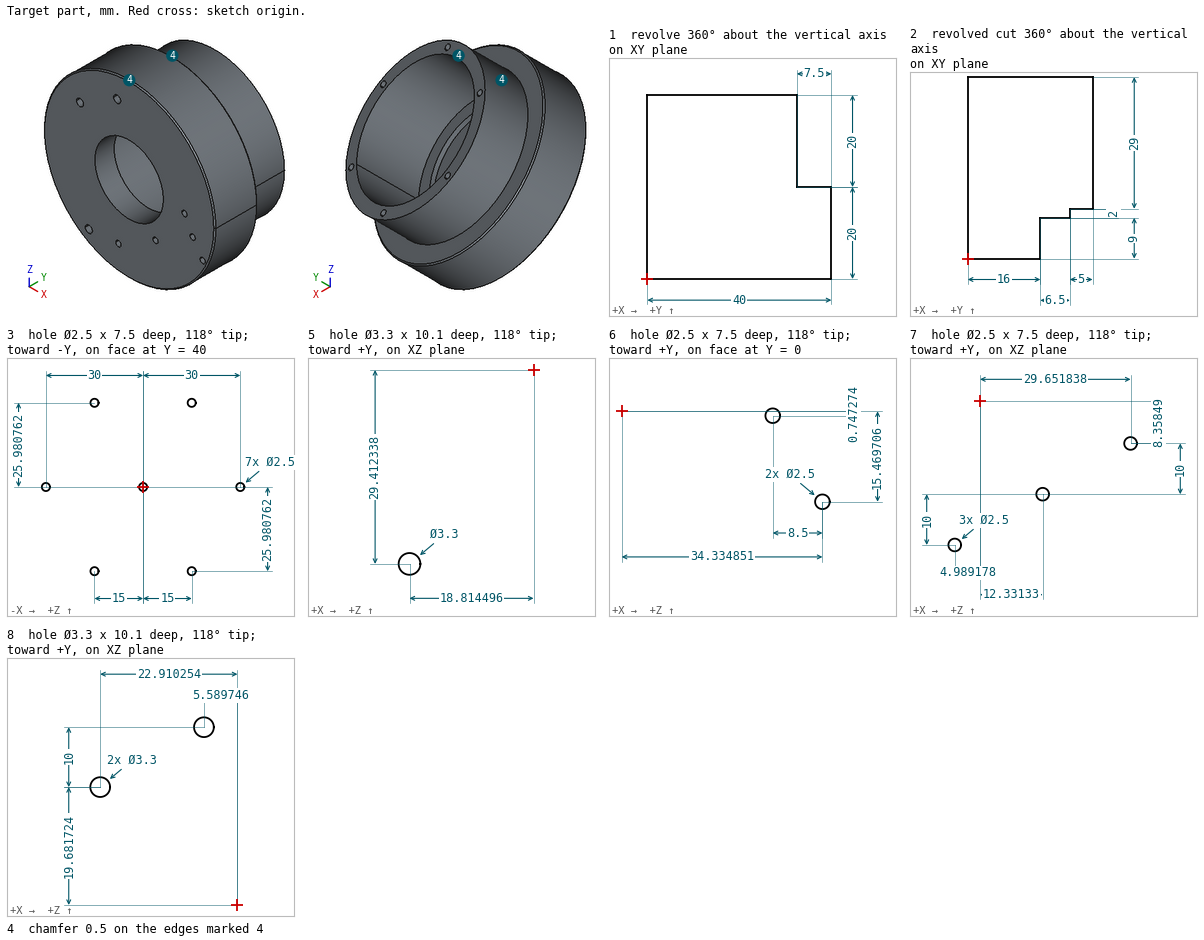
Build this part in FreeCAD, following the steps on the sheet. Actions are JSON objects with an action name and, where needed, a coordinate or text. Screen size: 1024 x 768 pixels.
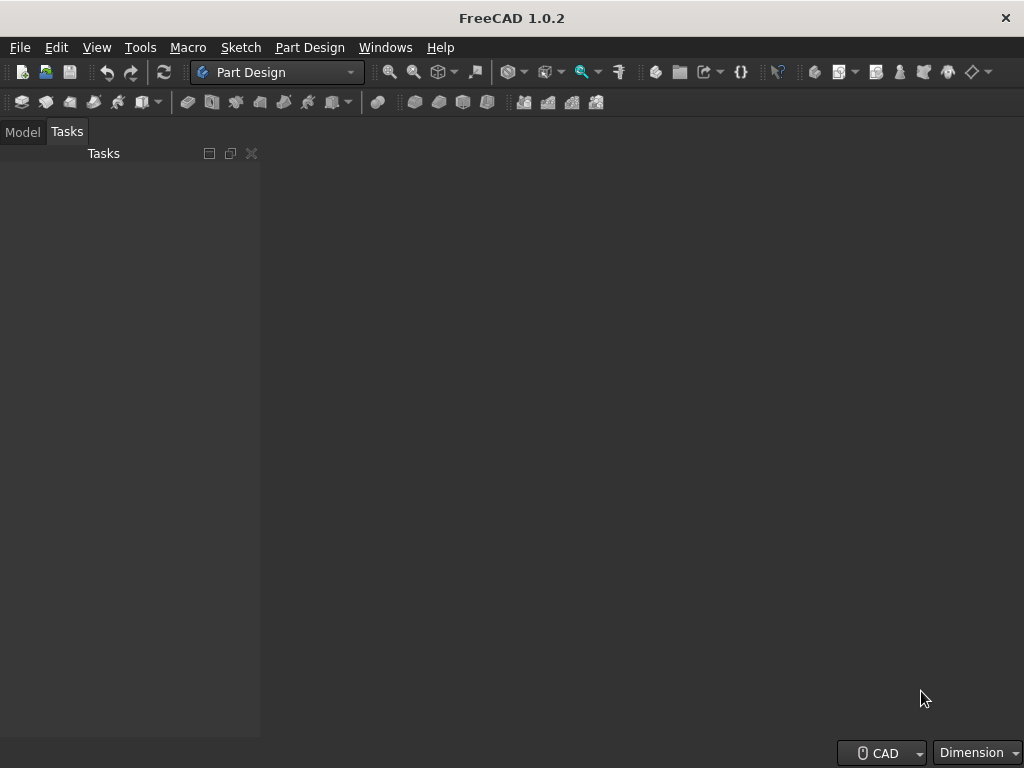
{"action": "left_click", "coordinate": [22, 72]}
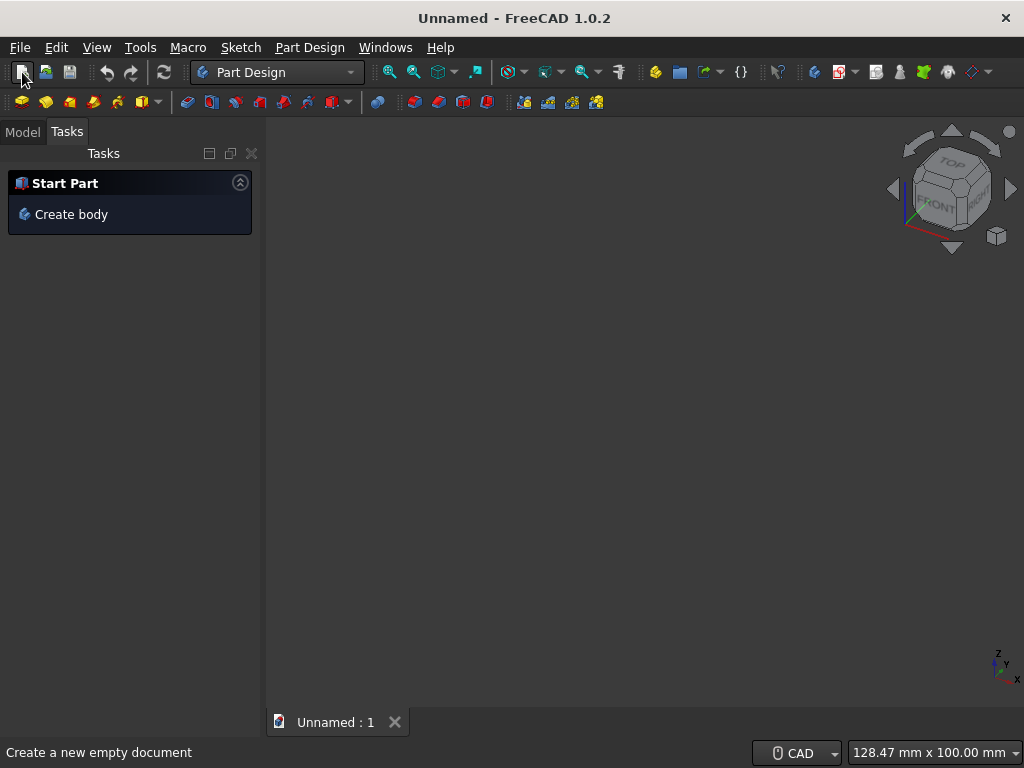
{"action": "left_click", "coordinate": [840, 72]}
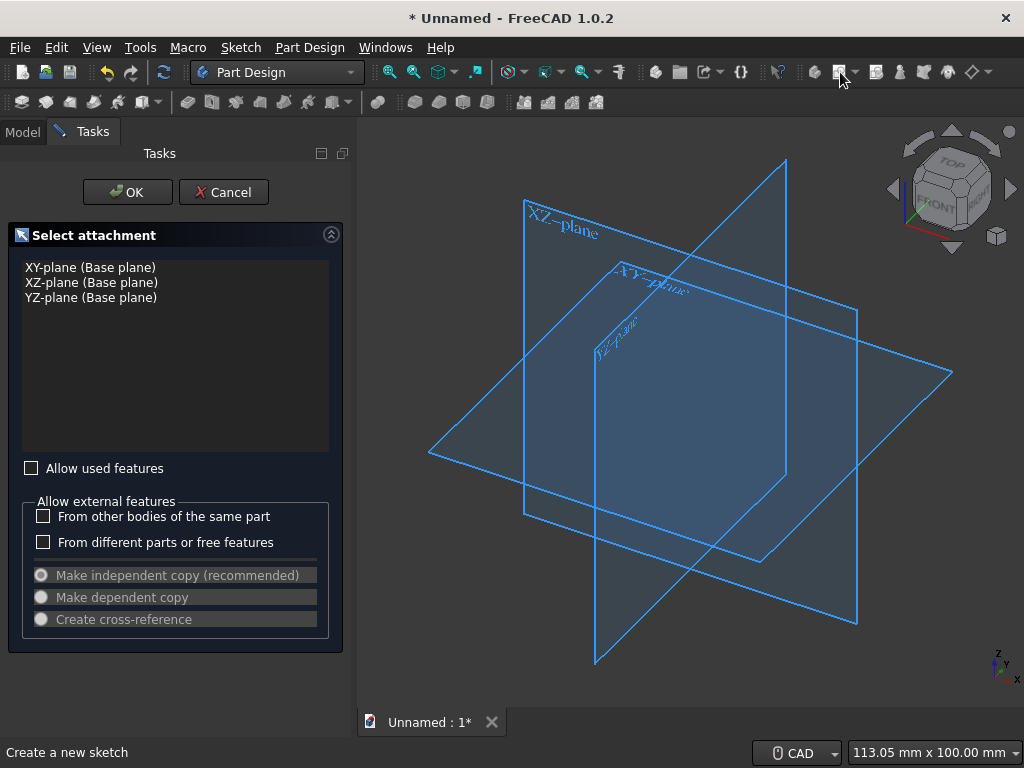
{"action": "left_click", "coordinate": [82, 268]}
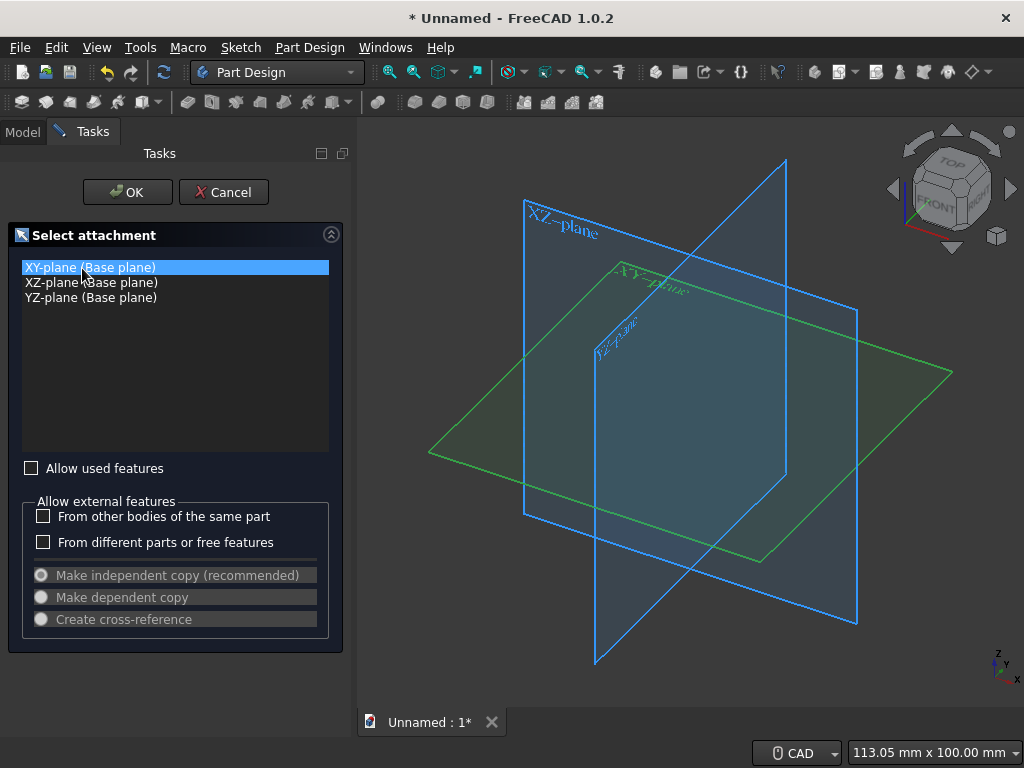
{"action": "left_click", "coordinate": [128, 192]}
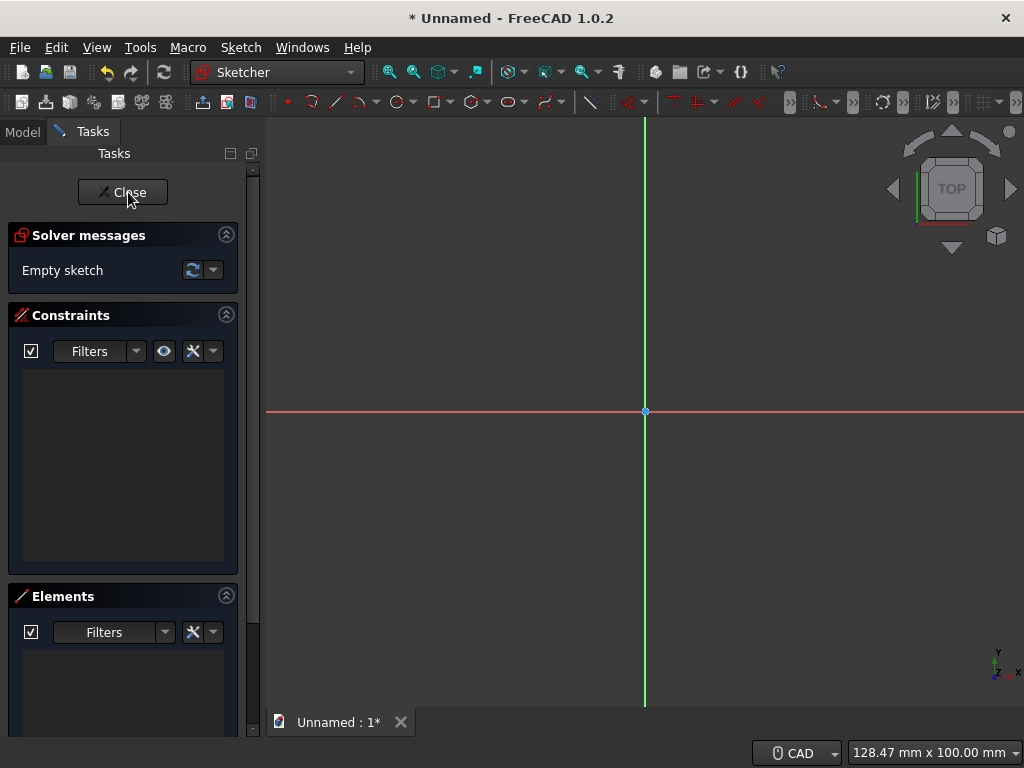
{"action": "scroll", "coordinate": [294, 679], "scroll_direction": "down", "scroll_amount": 1}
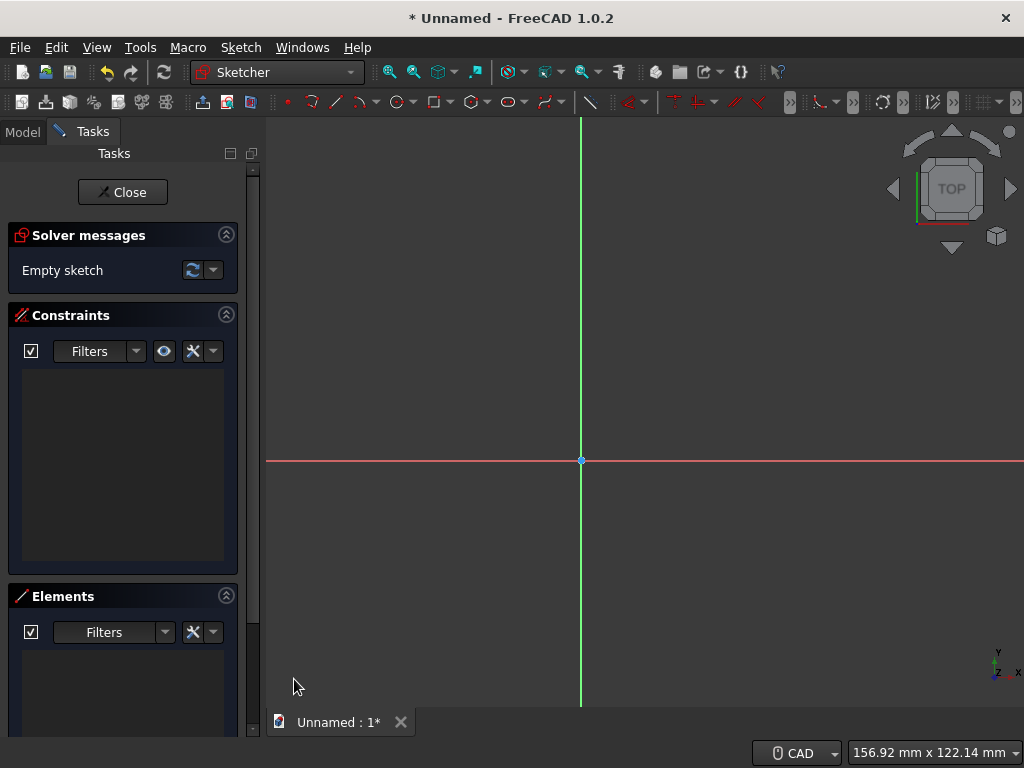
{"action": "scroll", "coordinate": [801, 306], "scroll_direction": "up", "scroll_amount": 3}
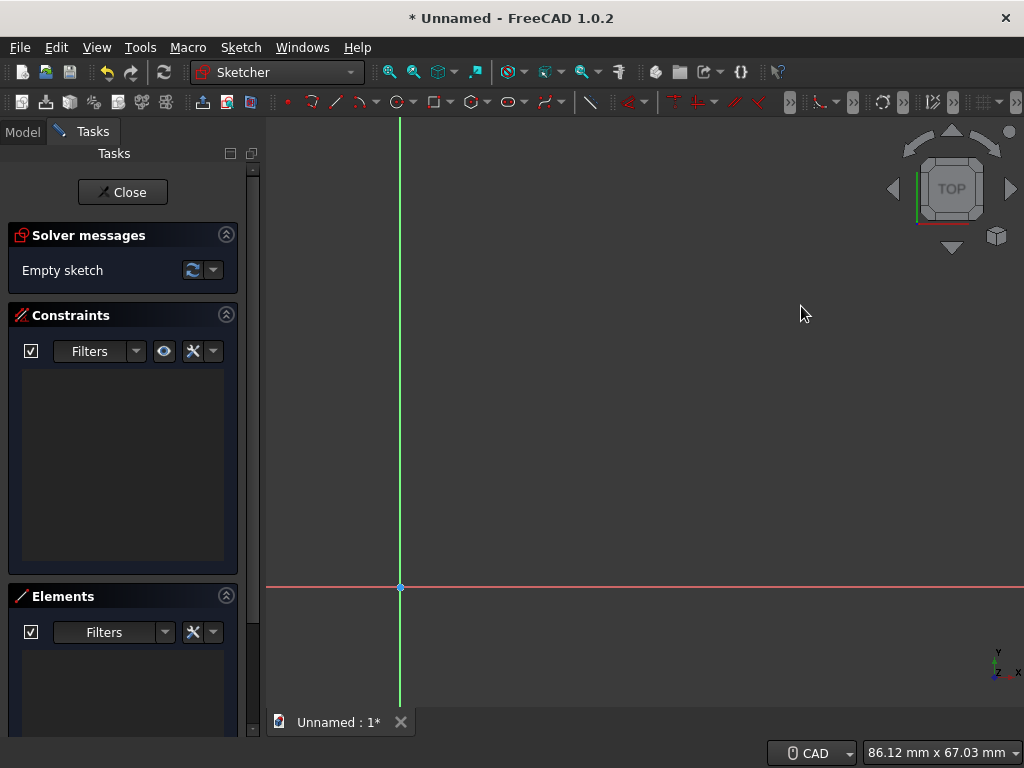
{"action": "left_click", "coordinate": [312, 102]}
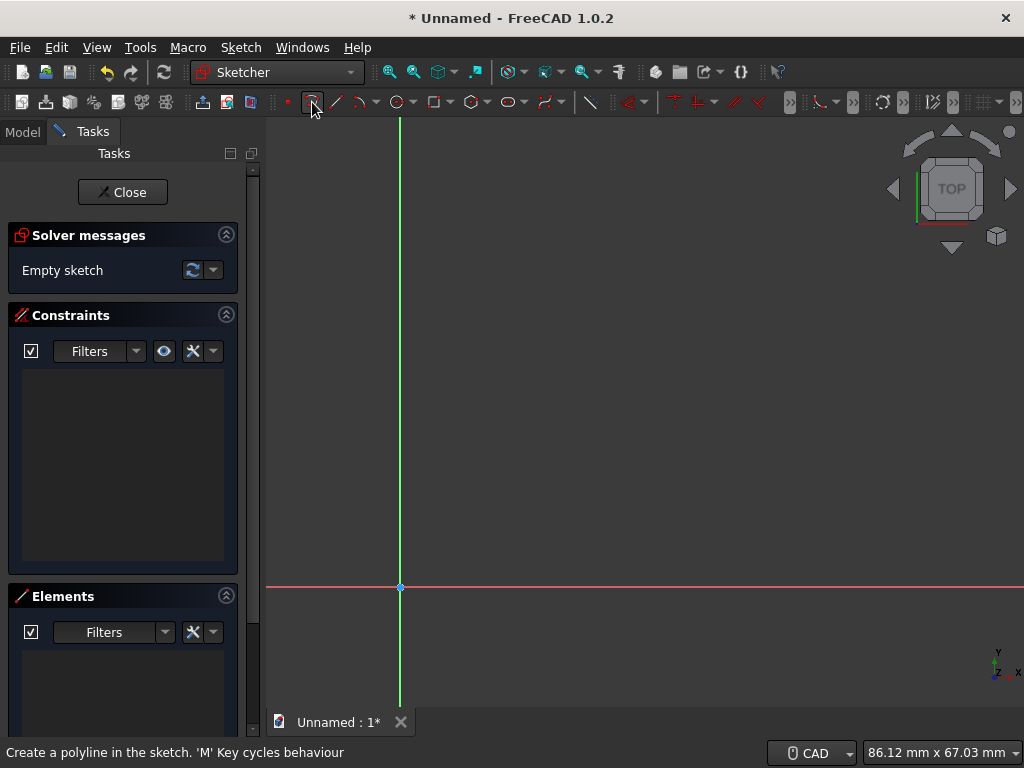
{"action": "left_click", "coordinate": [400, 587]}
{"action": "left_click", "coordinate": [752, 578]}
{"action": "left_click", "coordinate": [752, 411]}
{"action": "left_click", "coordinate": [686, 411]}
{"action": "left_click", "coordinate": [686, 235]}
{"action": "left_click", "coordinate": [409, 235]}
{"action": "left_click", "coordinate": [400, 587]}
{"action": "key", "text": "Escape"}
{"action": "key", "text": "Escape"}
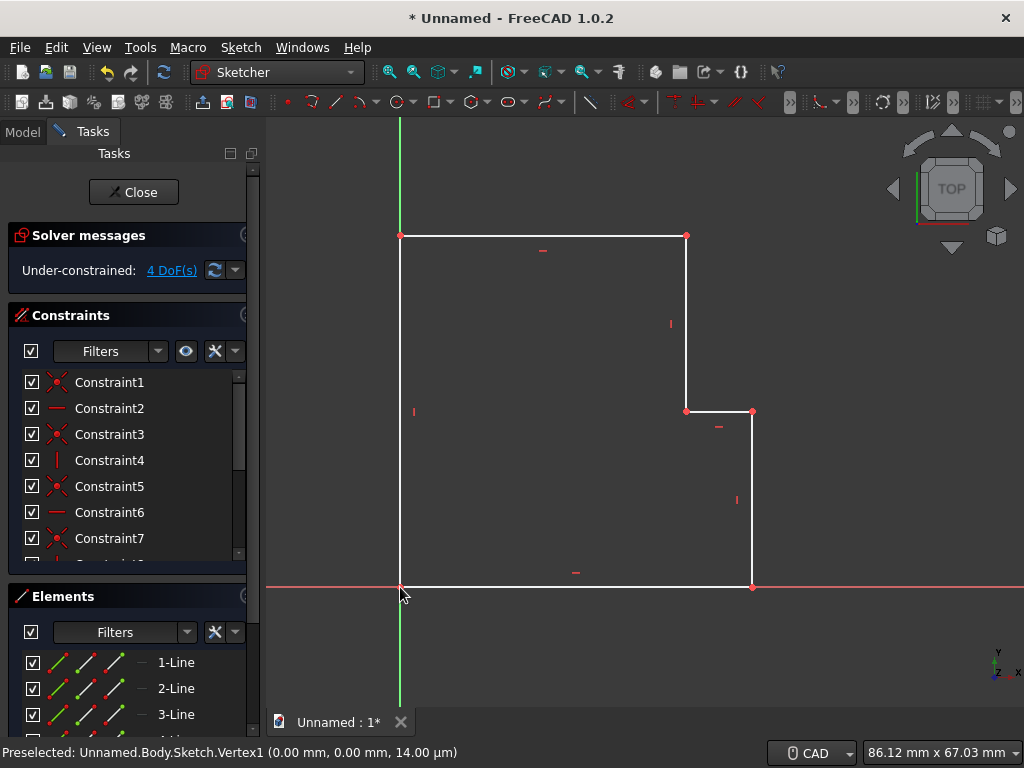
{"action": "left_click", "coordinate": [628, 102]}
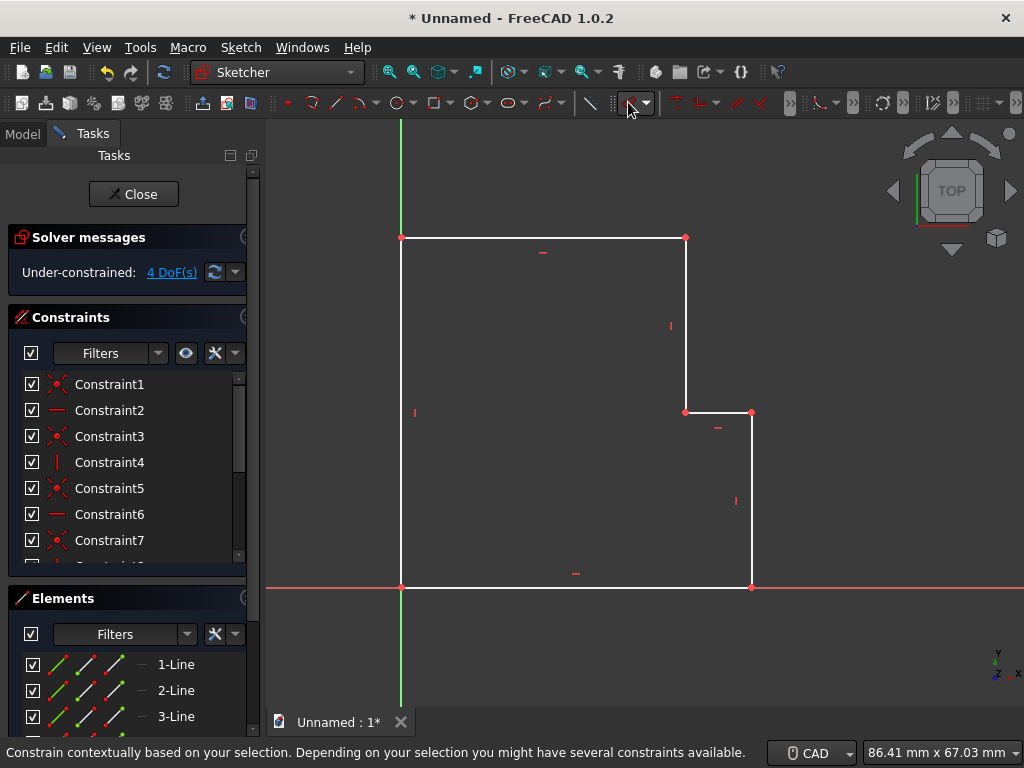
{"action": "left_click", "coordinate": [506, 588]}
{"action": "left_click", "coordinate": [576, 622]}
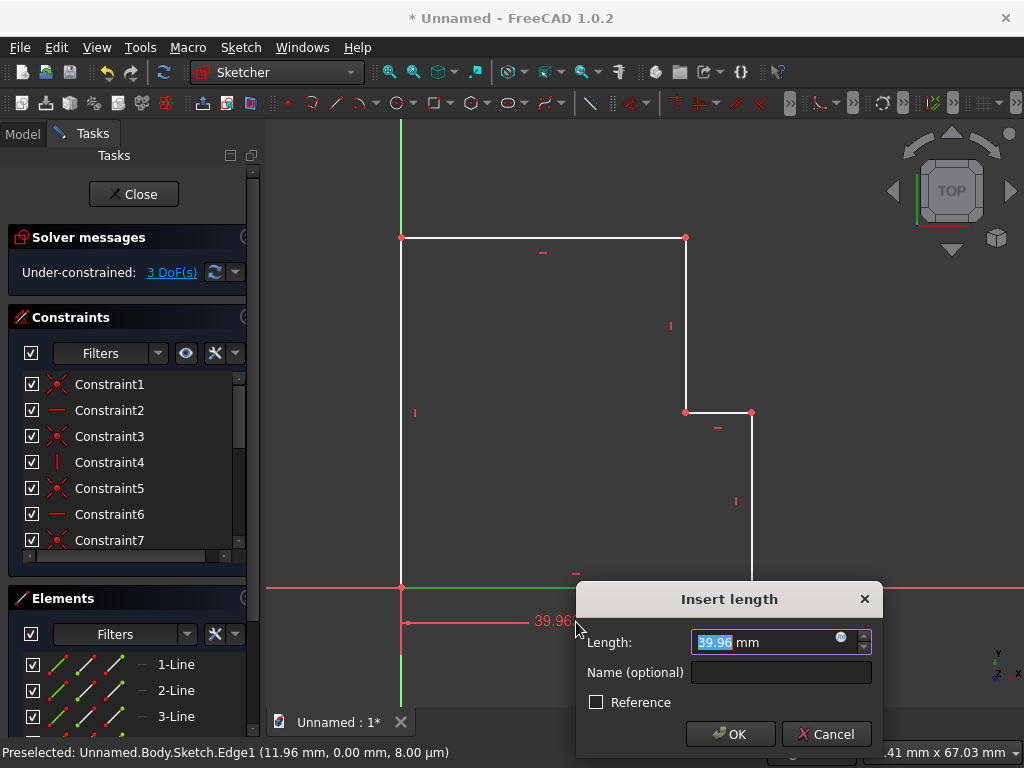
{"action": "type", "text": "40"}
{"action": "key", "text": "Return"}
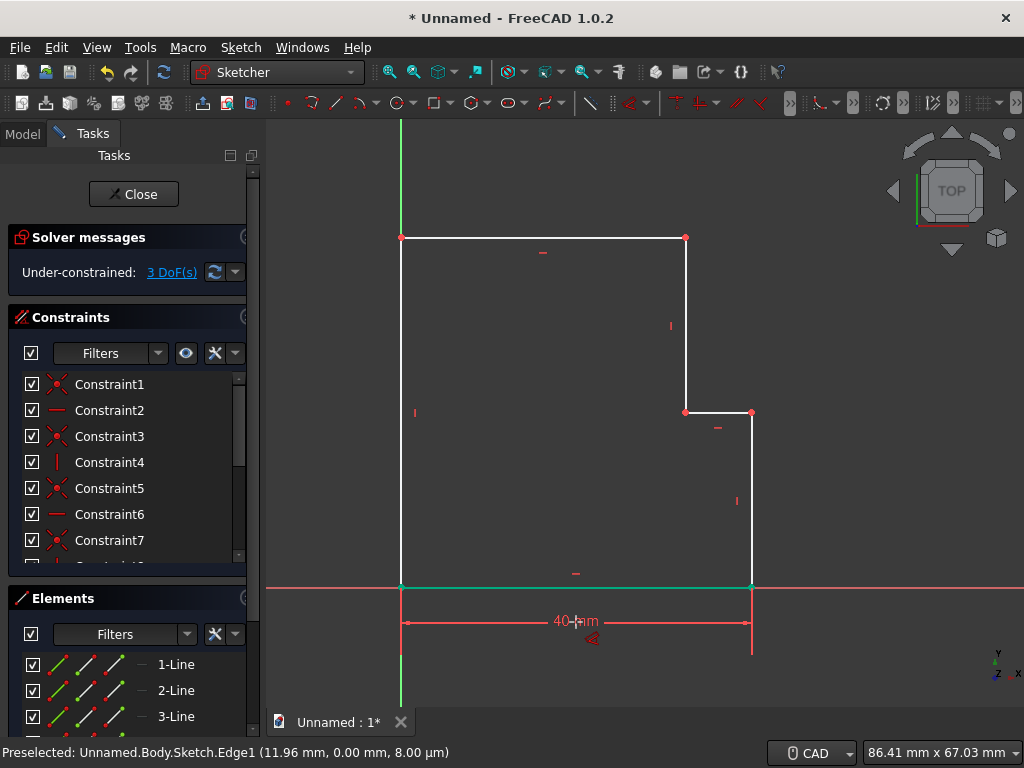
{"action": "left_click", "coordinate": [752, 535]}
{"action": "left_click", "coordinate": [786, 500]}